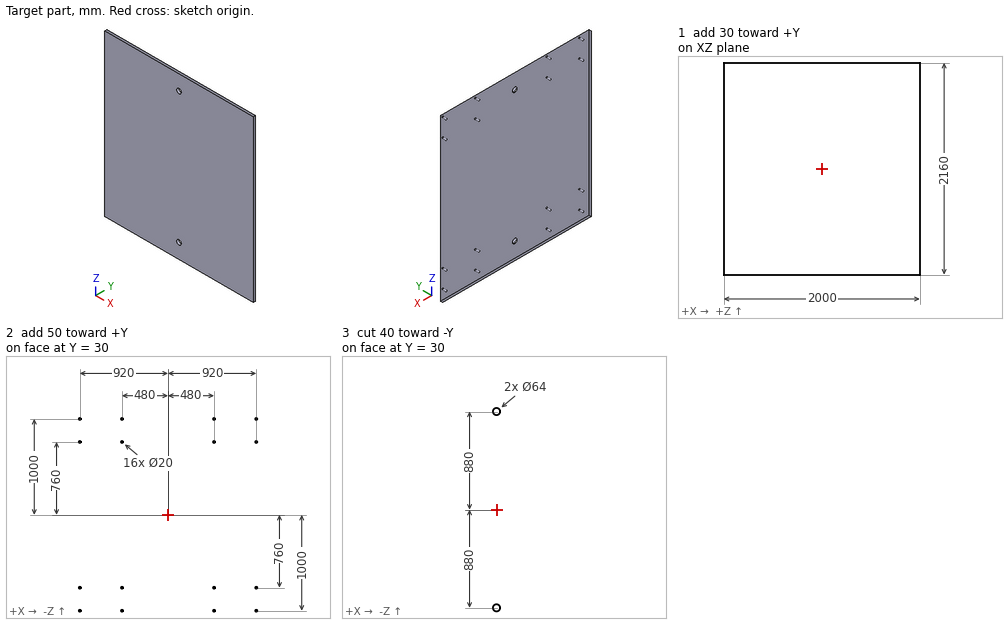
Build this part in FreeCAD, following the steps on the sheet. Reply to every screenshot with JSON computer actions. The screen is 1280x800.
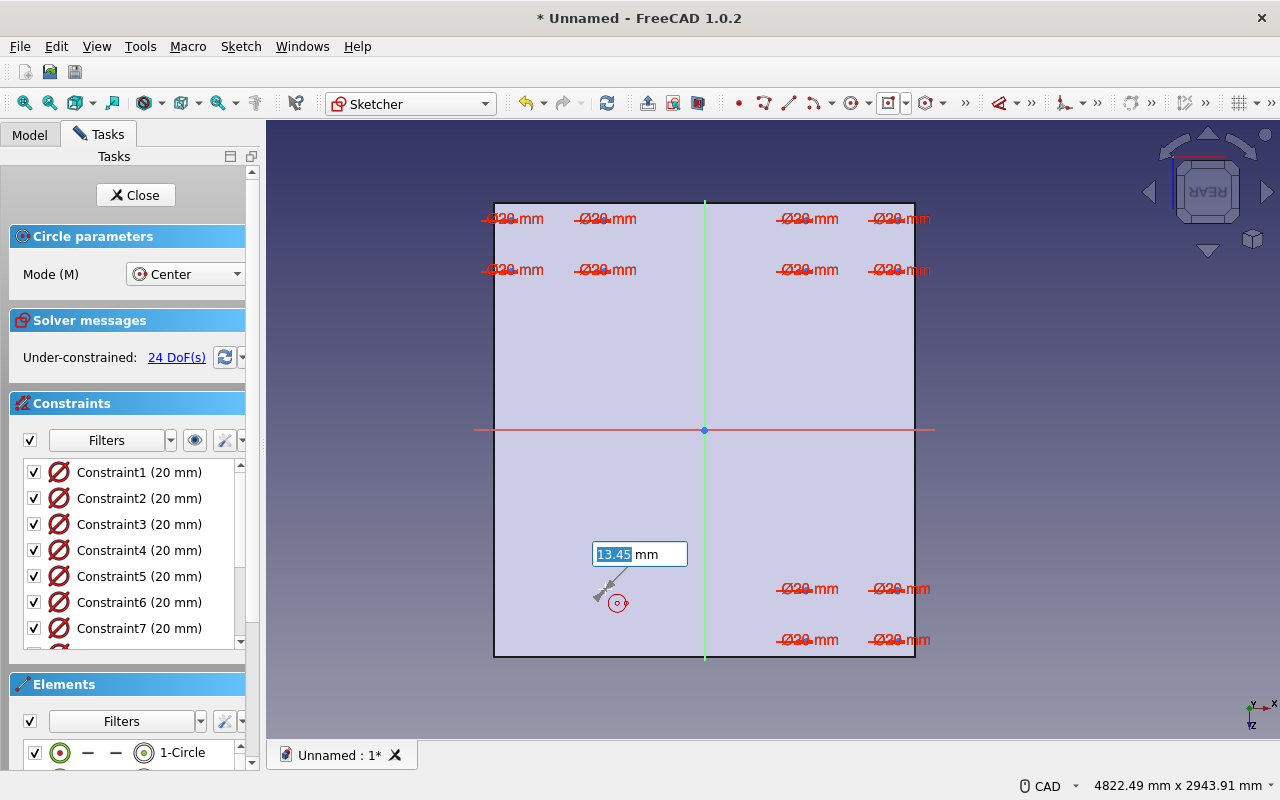
{"action": "type", "text": "20"}
{"action": "key", "text": "Return"}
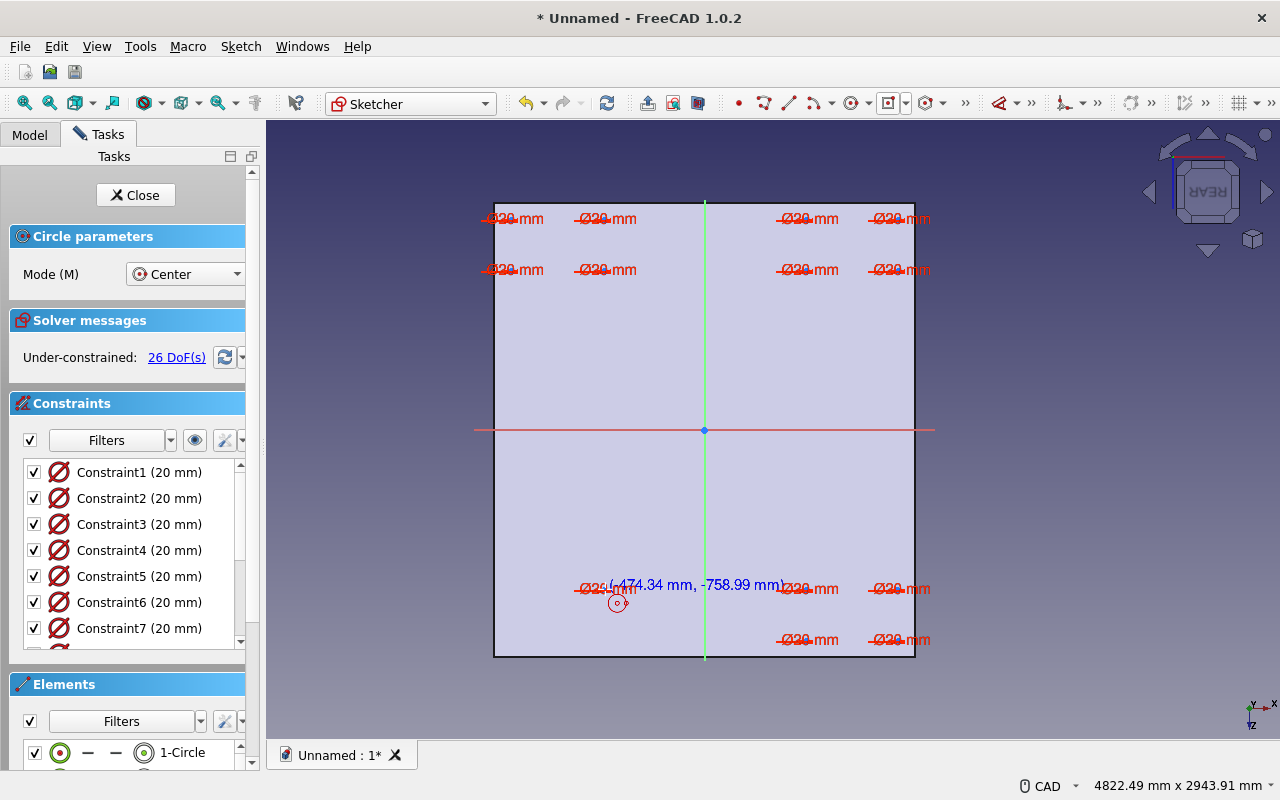
{"action": "scroll", "coordinate": [604, 641], "scroll_direction": "up", "scroll_amount": 12}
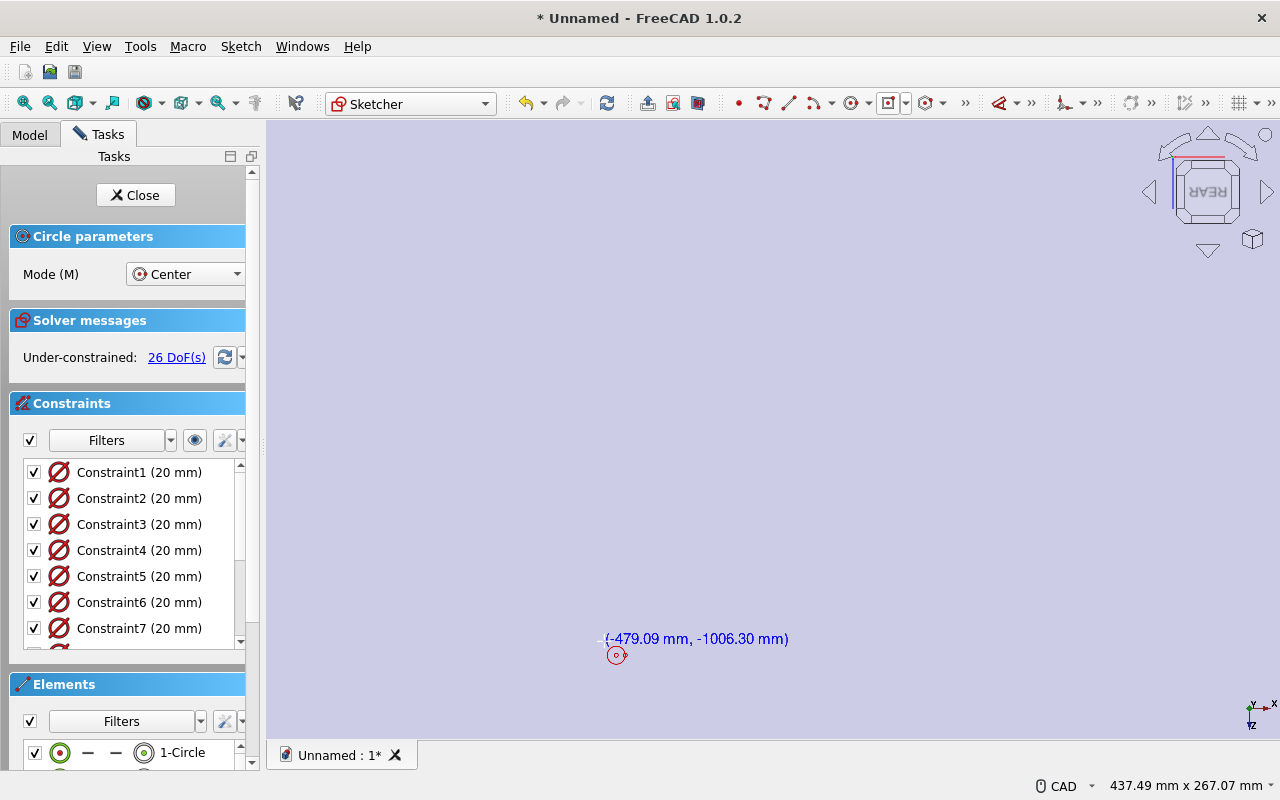
{"action": "scroll", "coordinate": [604, 641], "scroll_direction": "down", "scroll_amount": 12}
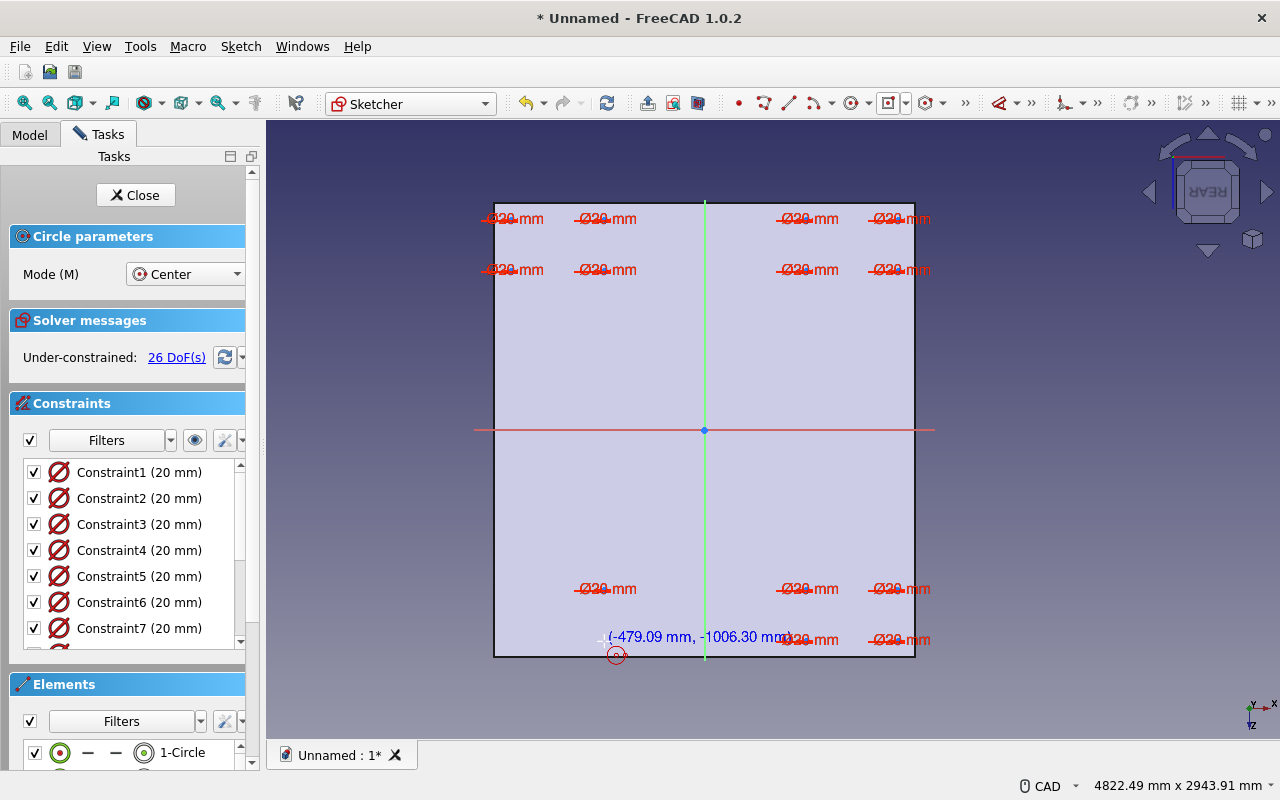
{"action": "left_click", "coordinate": [604, 641]}
{"action": "mouse_move", "coordinate": [605, 639]}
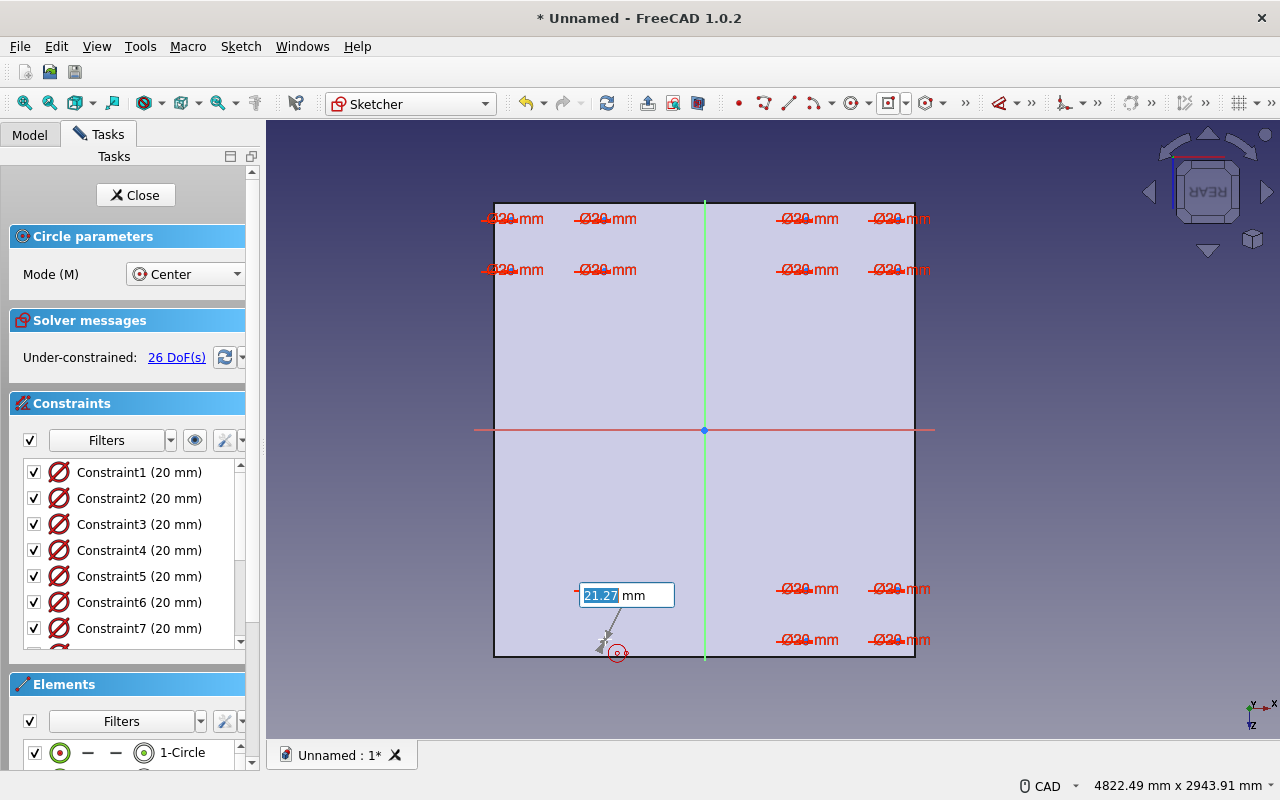
{"action": "type", "text": "20"}
{"action": "key", "text": "Return"}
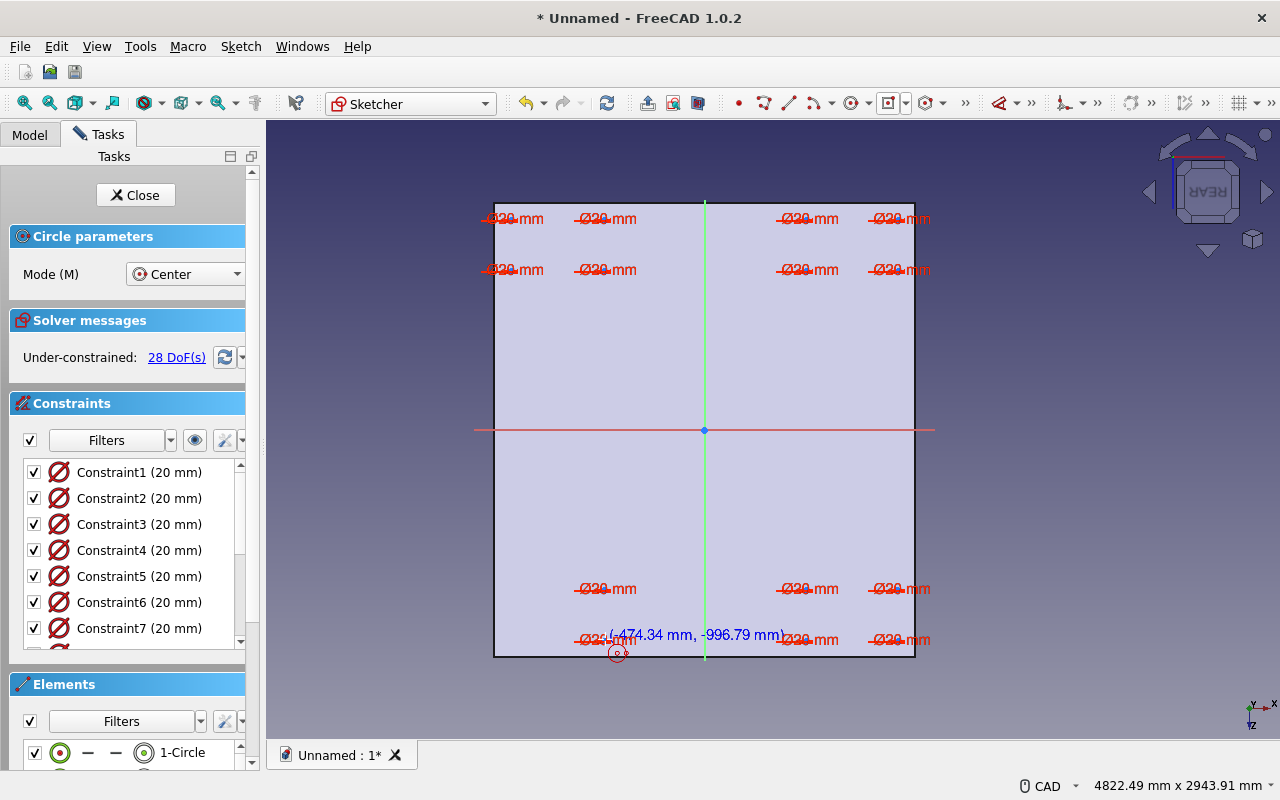
{"action": "scroll", "coordinate": [511, 590], "scroll_direction": "up", "scroll_amount": 12}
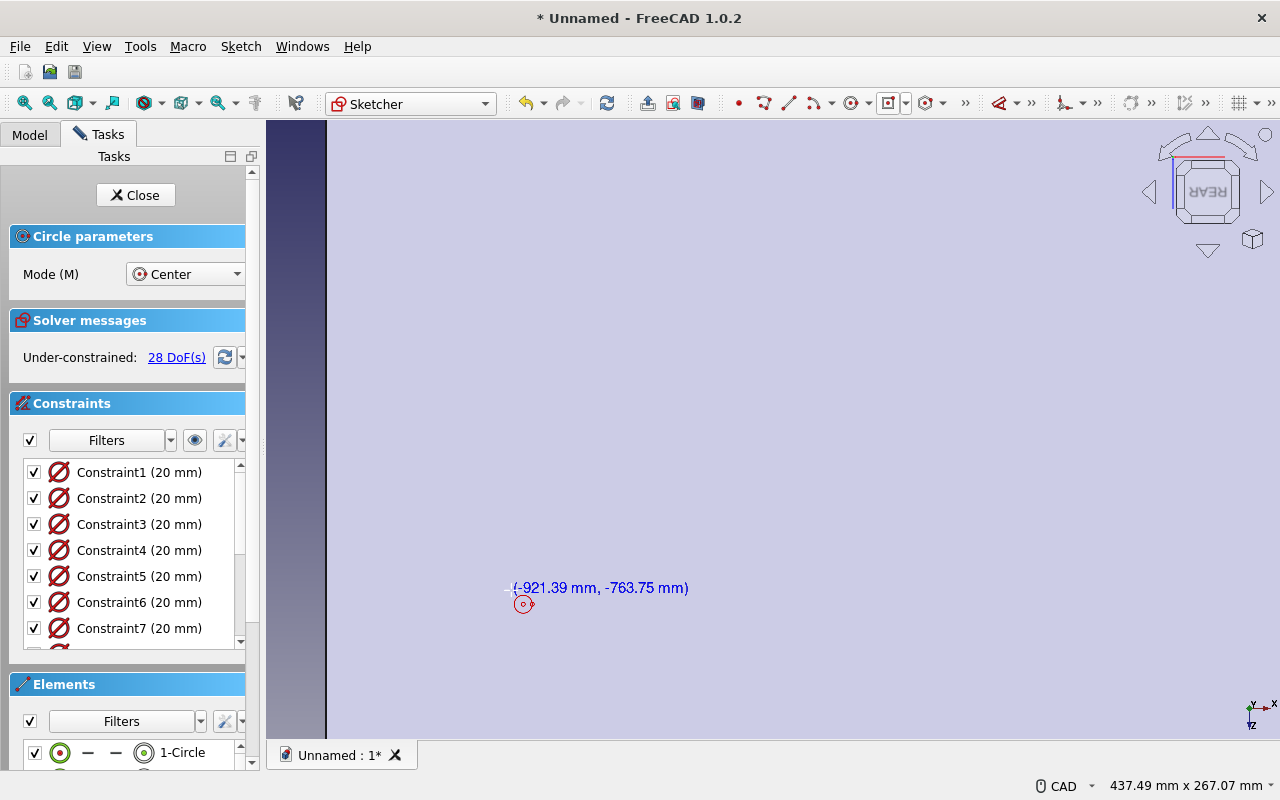
{"action": "scroll", "coordinate": [511, 590], "scroll_direction": "down", "scroll_amount": 12}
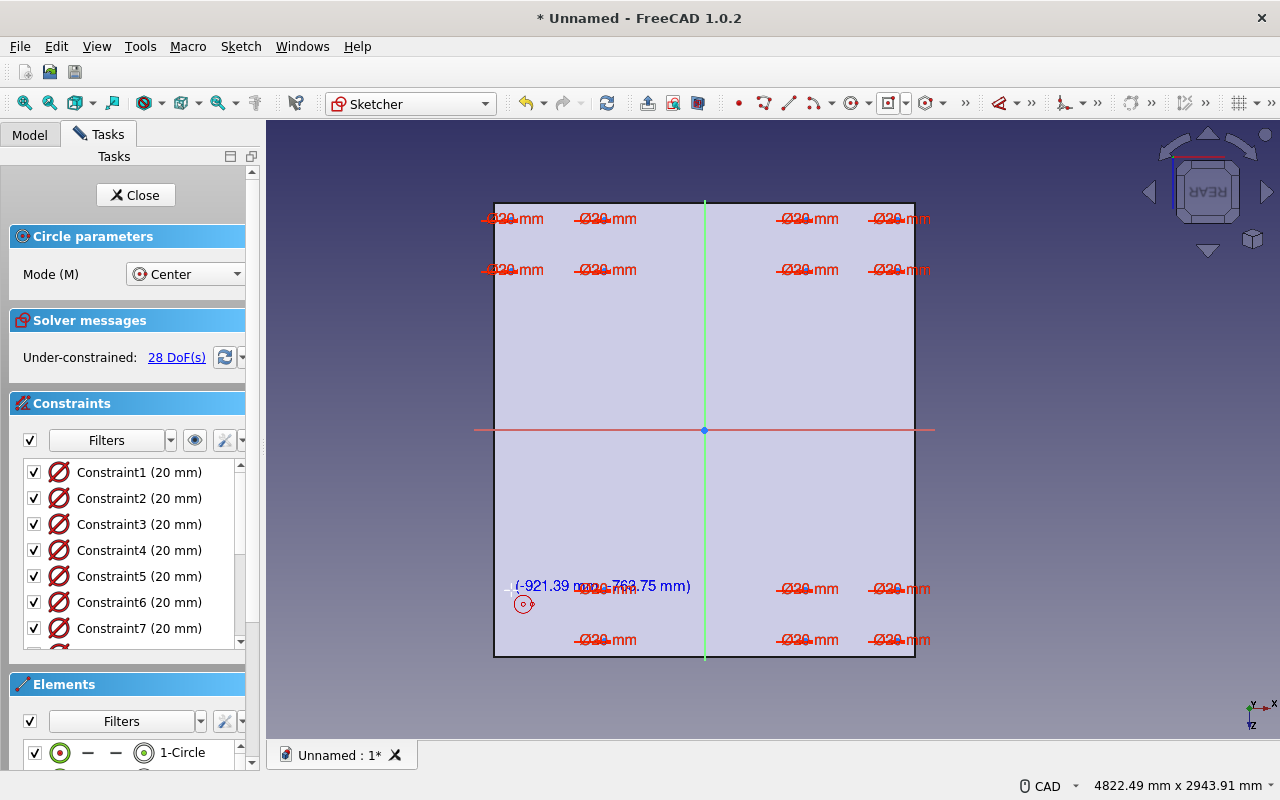
{"action": "left_click", "coordinate": [511, 590]}
{"action": "mouse_move", "coordinate": [513, 589]}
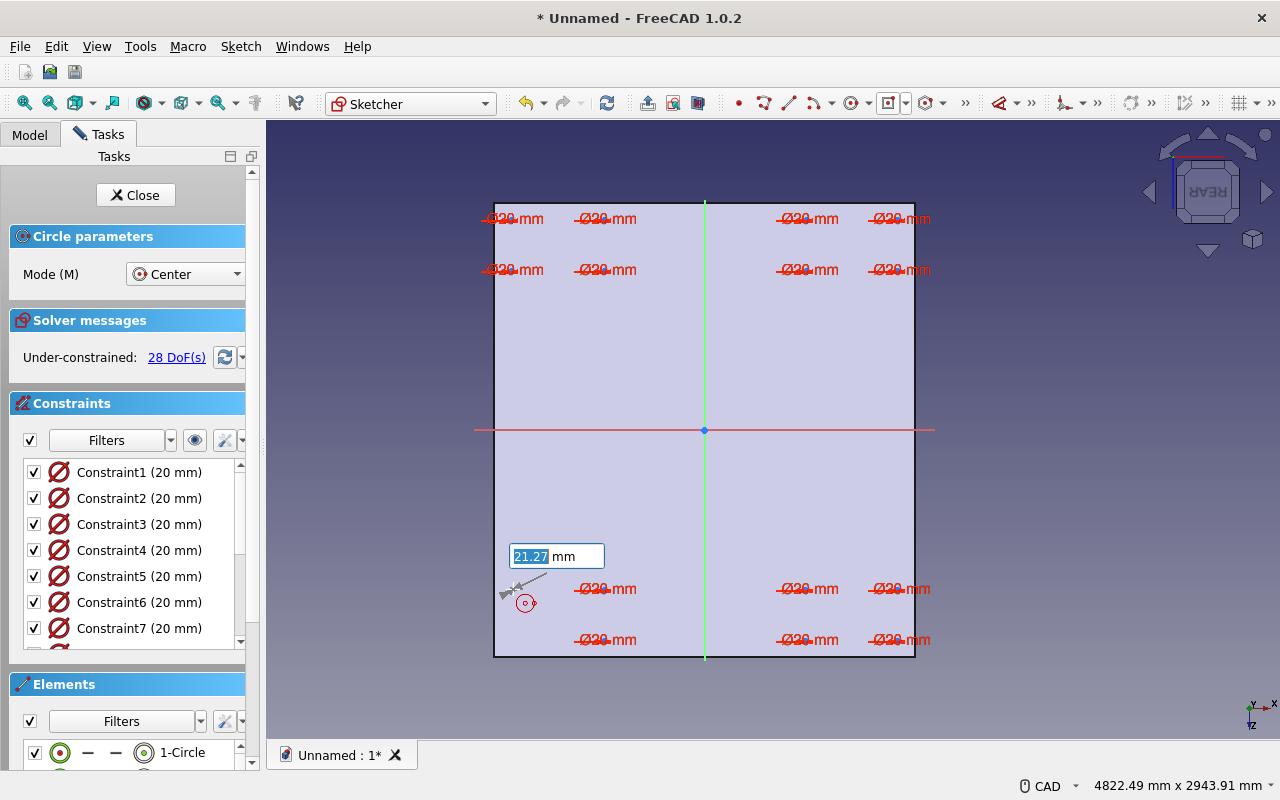
{"action": "type", "text": "20"}
{"action": "key", "text": "Return"}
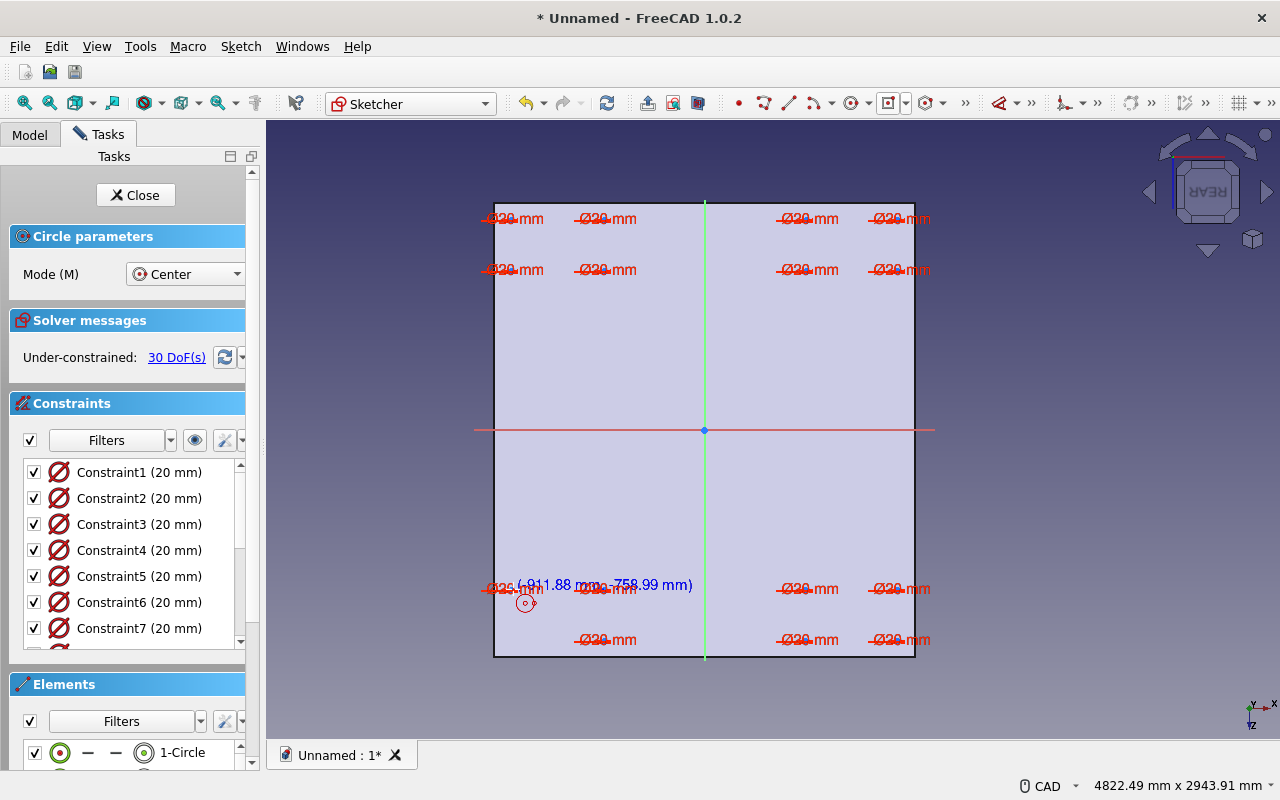
{"action": "scroll", "coordinate": [511, 641], "scroll_direction": "up", "scroll_amount": 12}